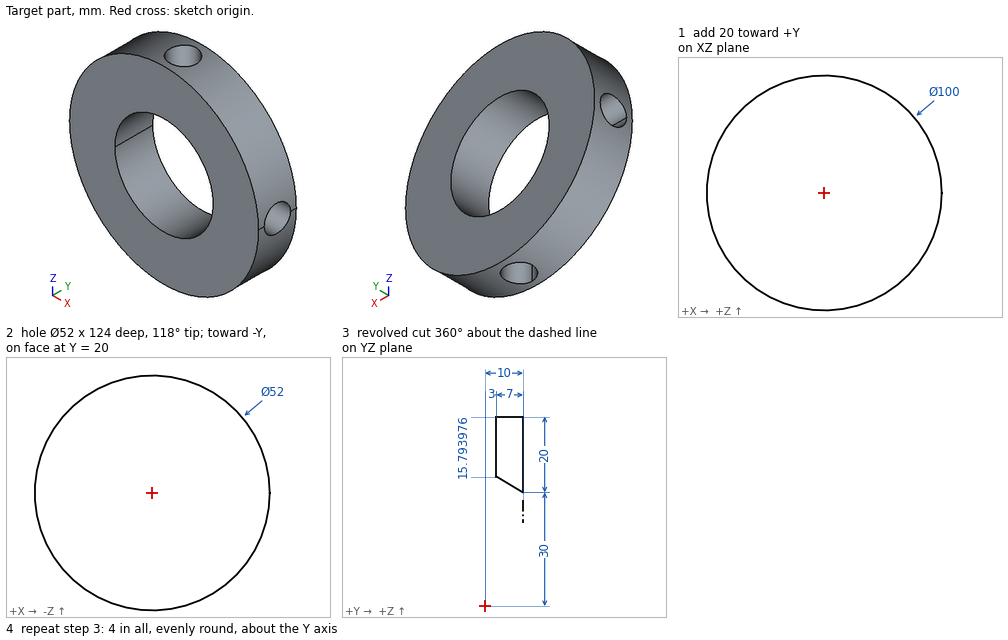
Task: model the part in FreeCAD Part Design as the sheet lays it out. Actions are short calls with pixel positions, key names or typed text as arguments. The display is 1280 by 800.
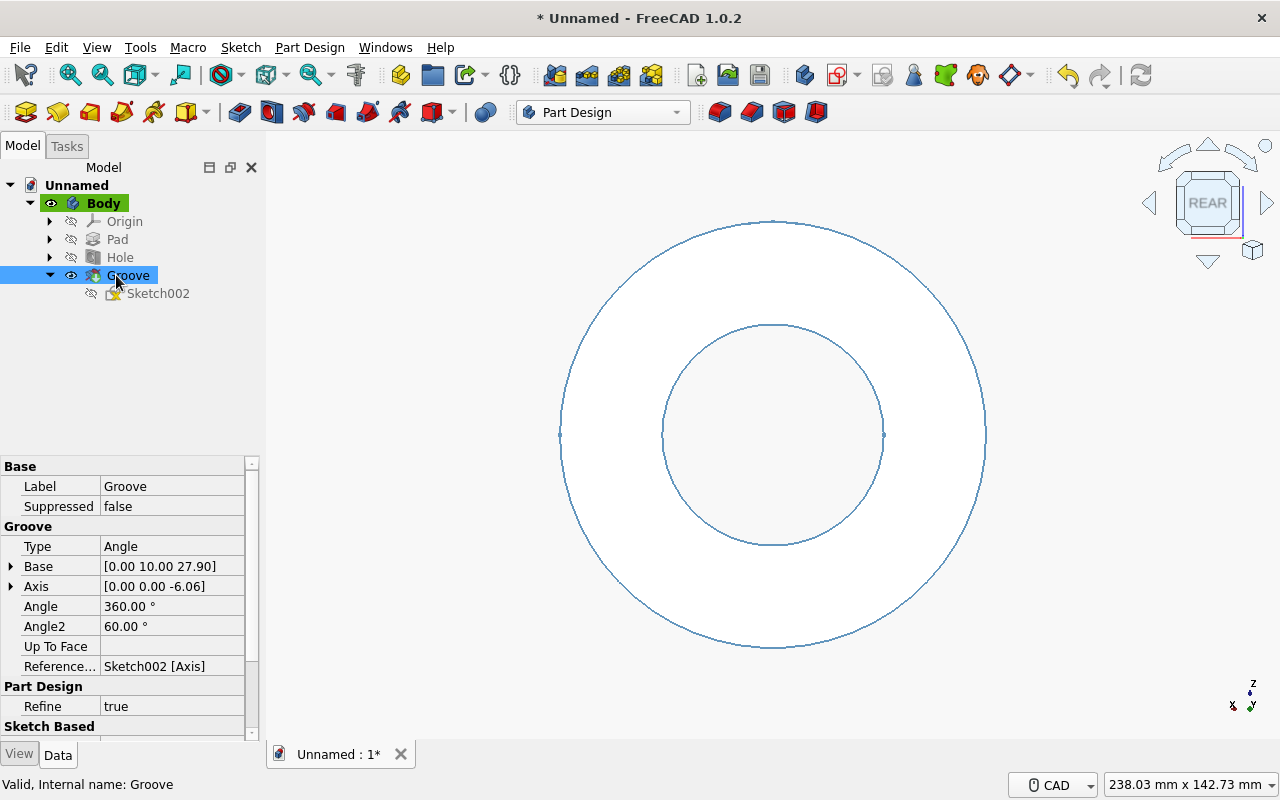
click(620, 76)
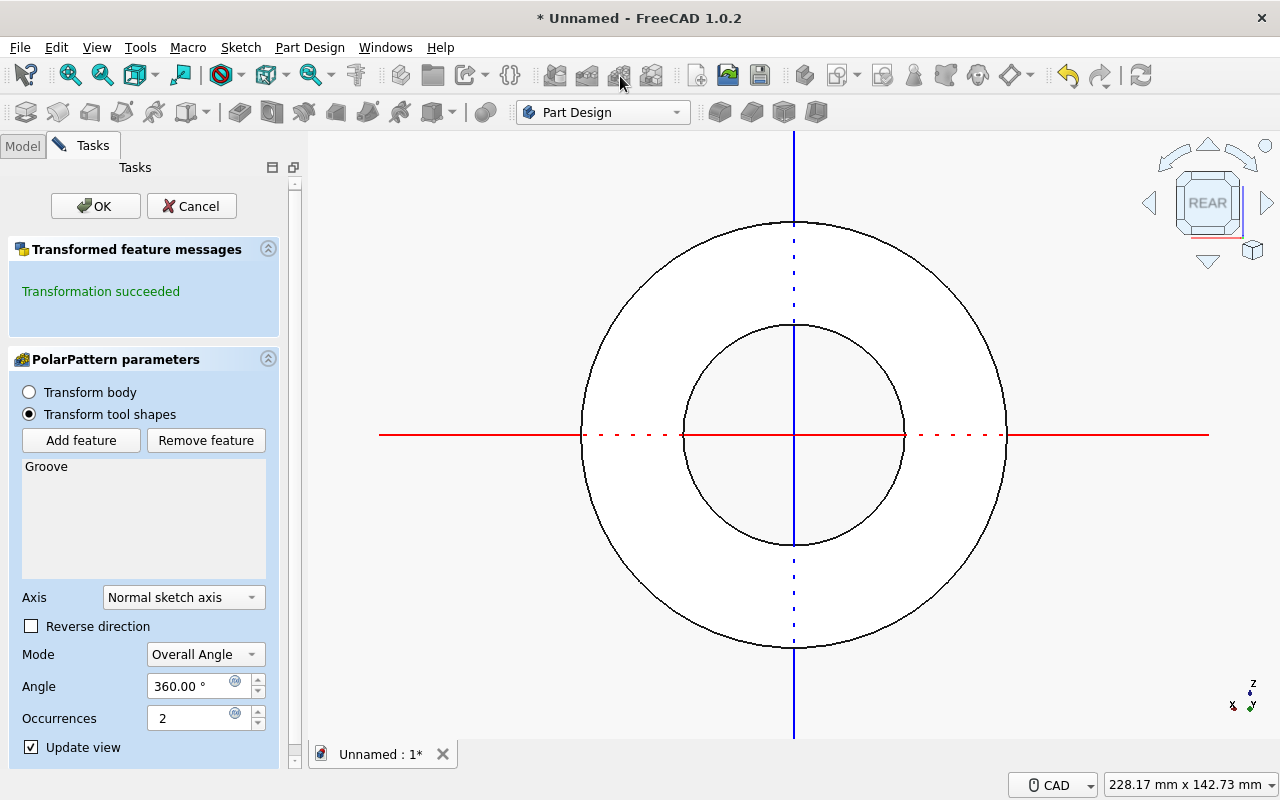
click(184, 598)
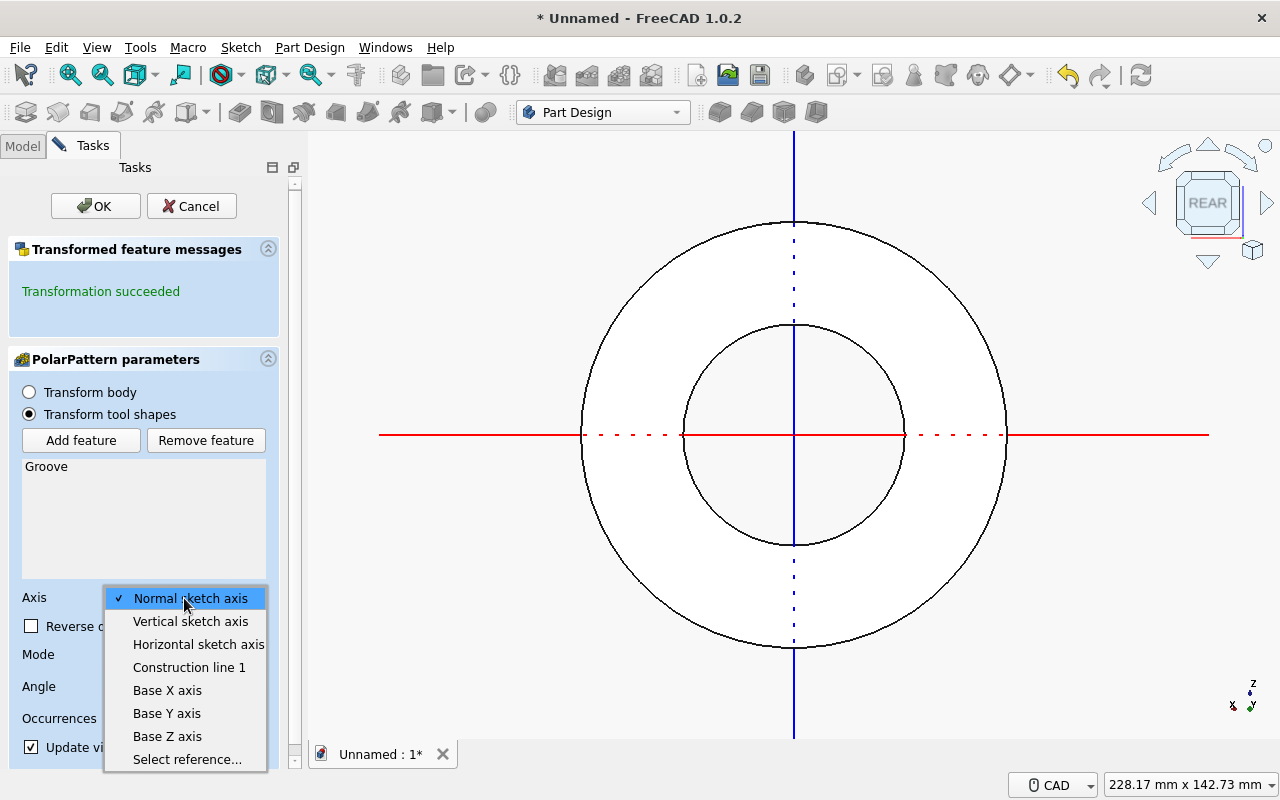
click(184, 714)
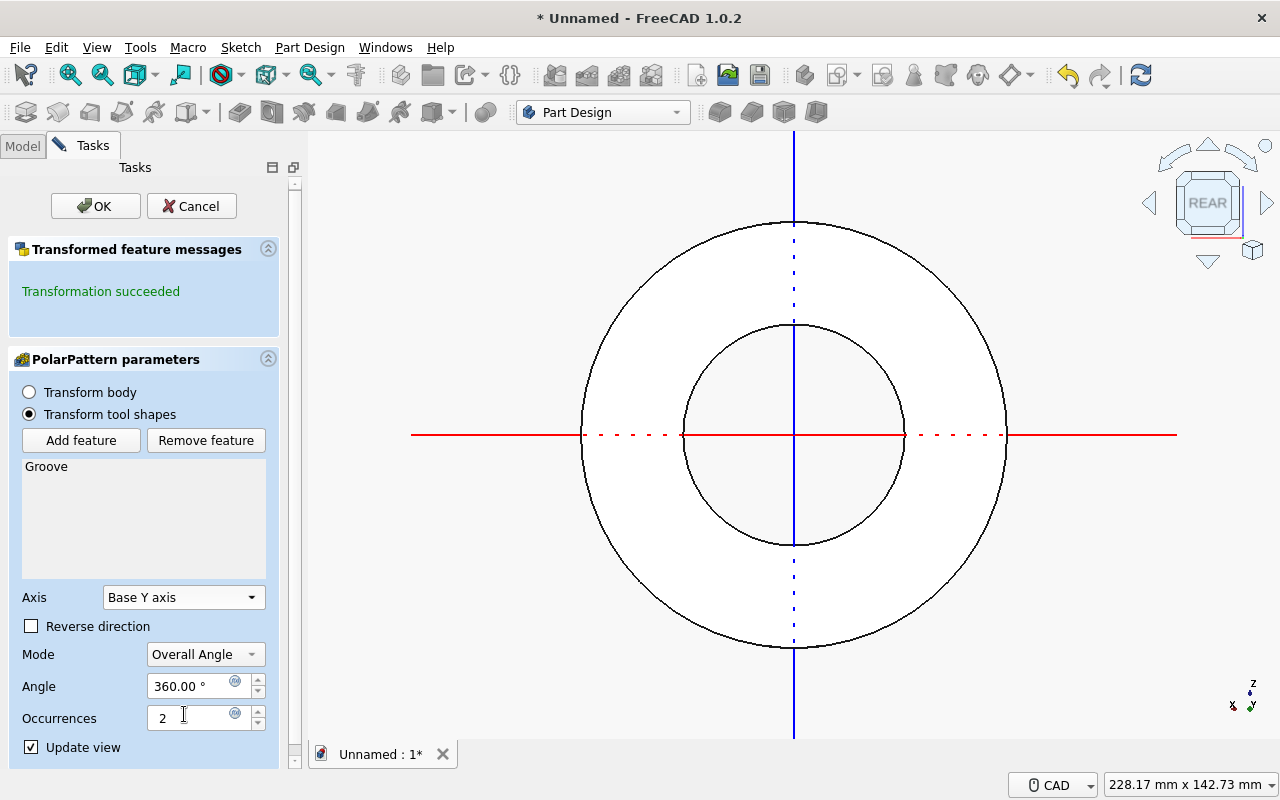
triple_click(198, 718)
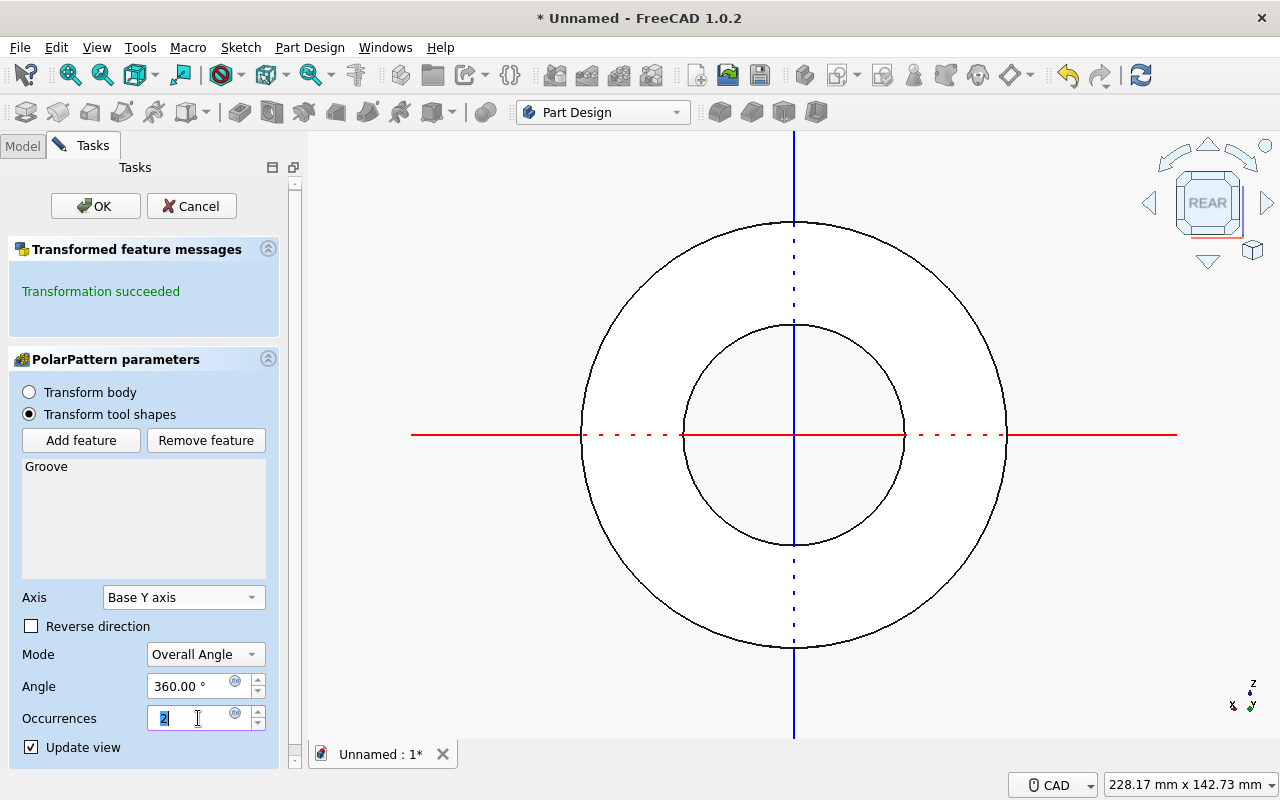
text(4)
key(Tab)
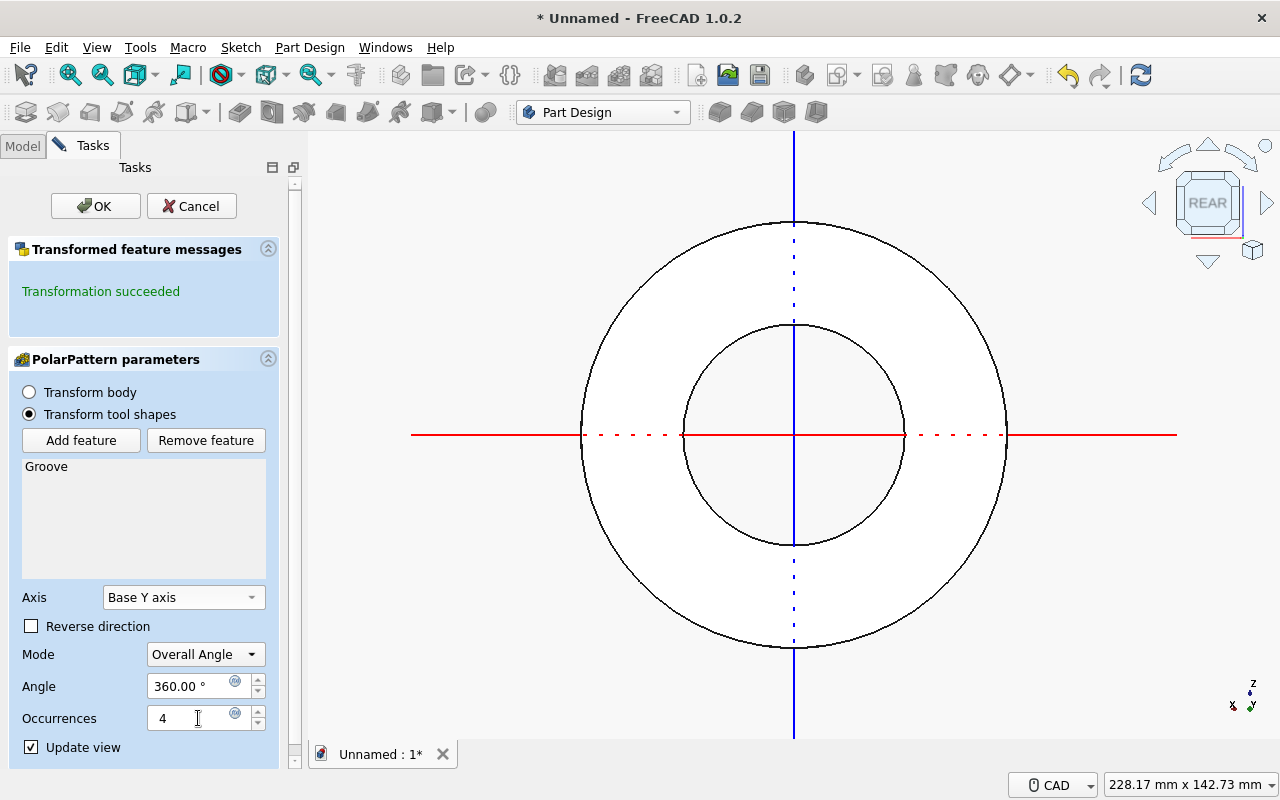
click(96, 206)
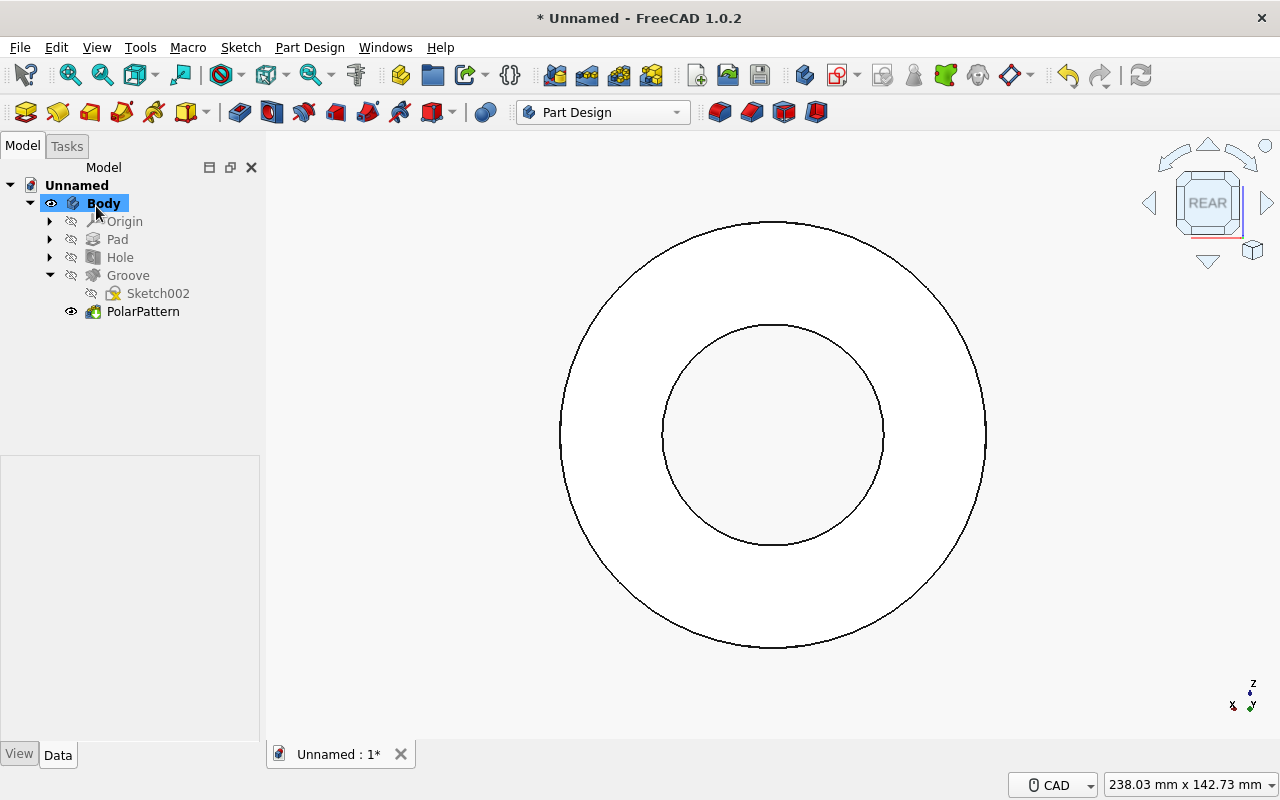
key(0)